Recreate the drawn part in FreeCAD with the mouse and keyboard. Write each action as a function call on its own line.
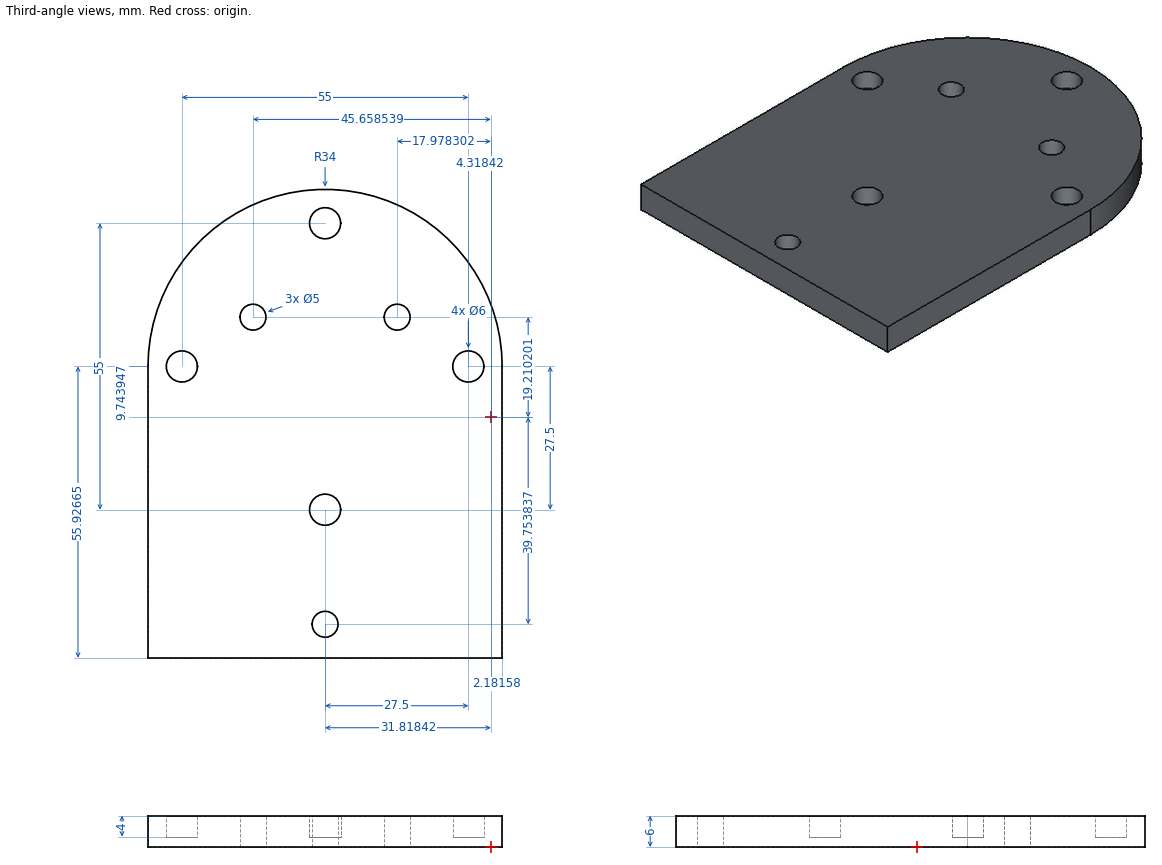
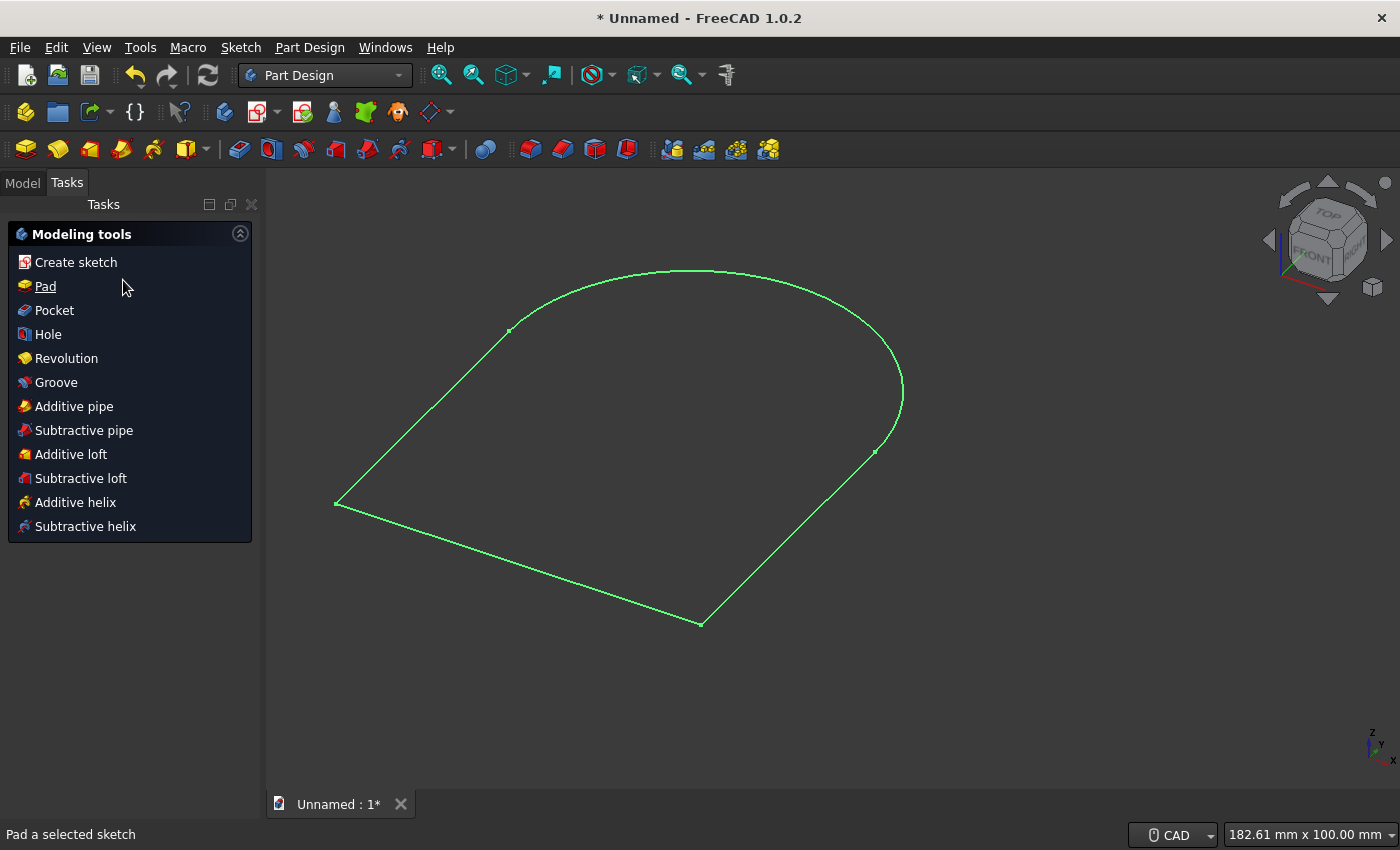
click(26, 150)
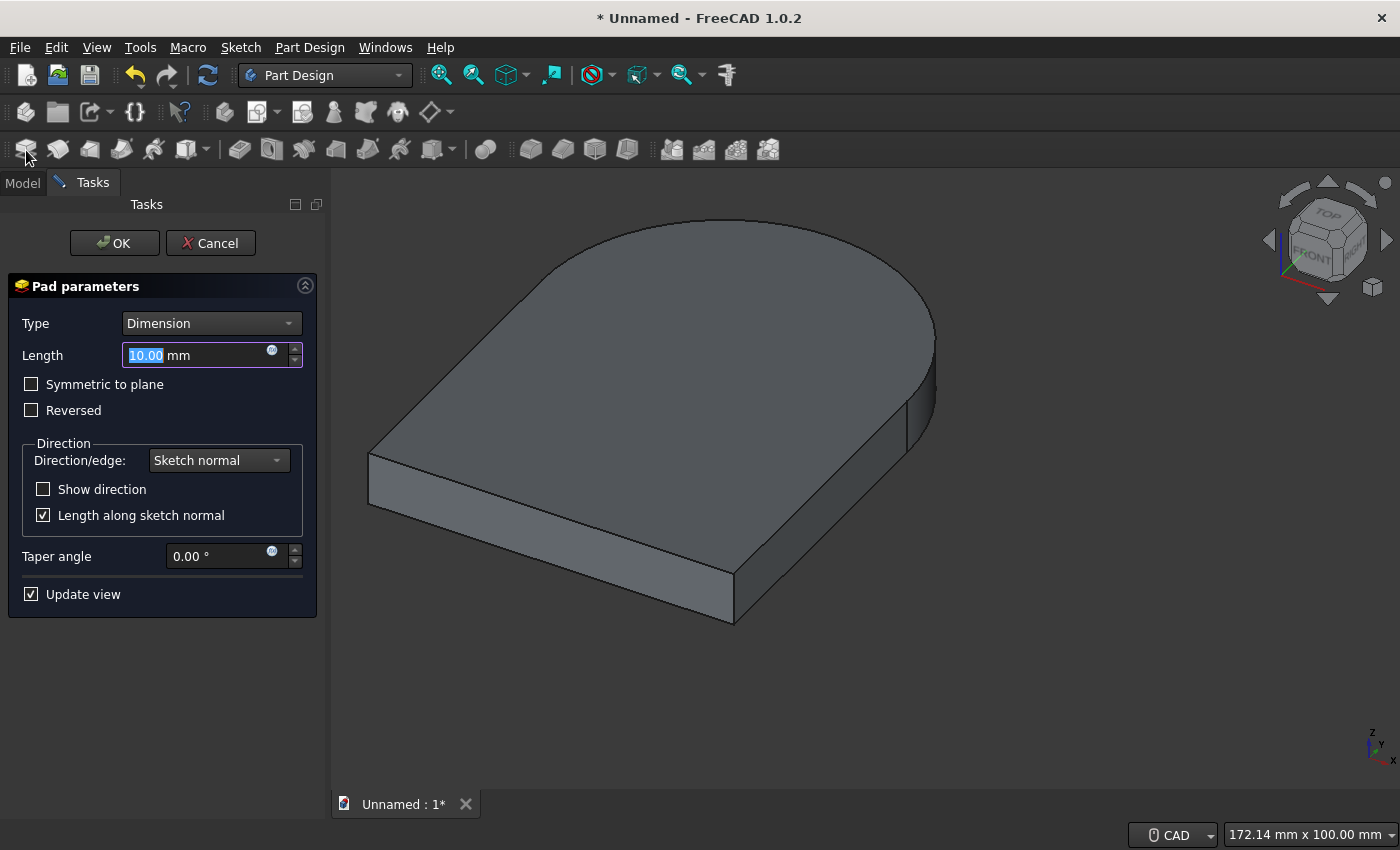
text(6)
key(Tab)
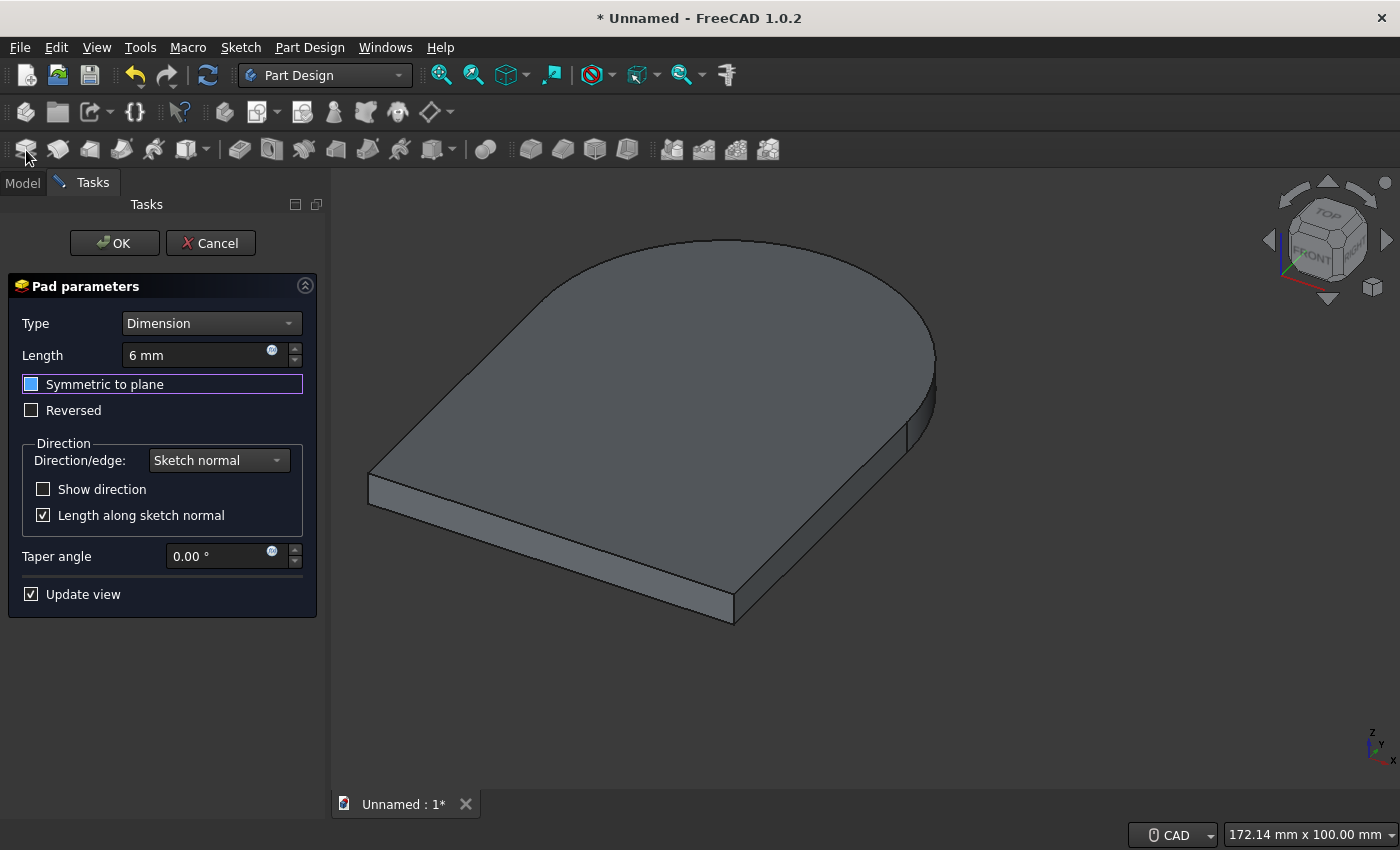
click(115, 243)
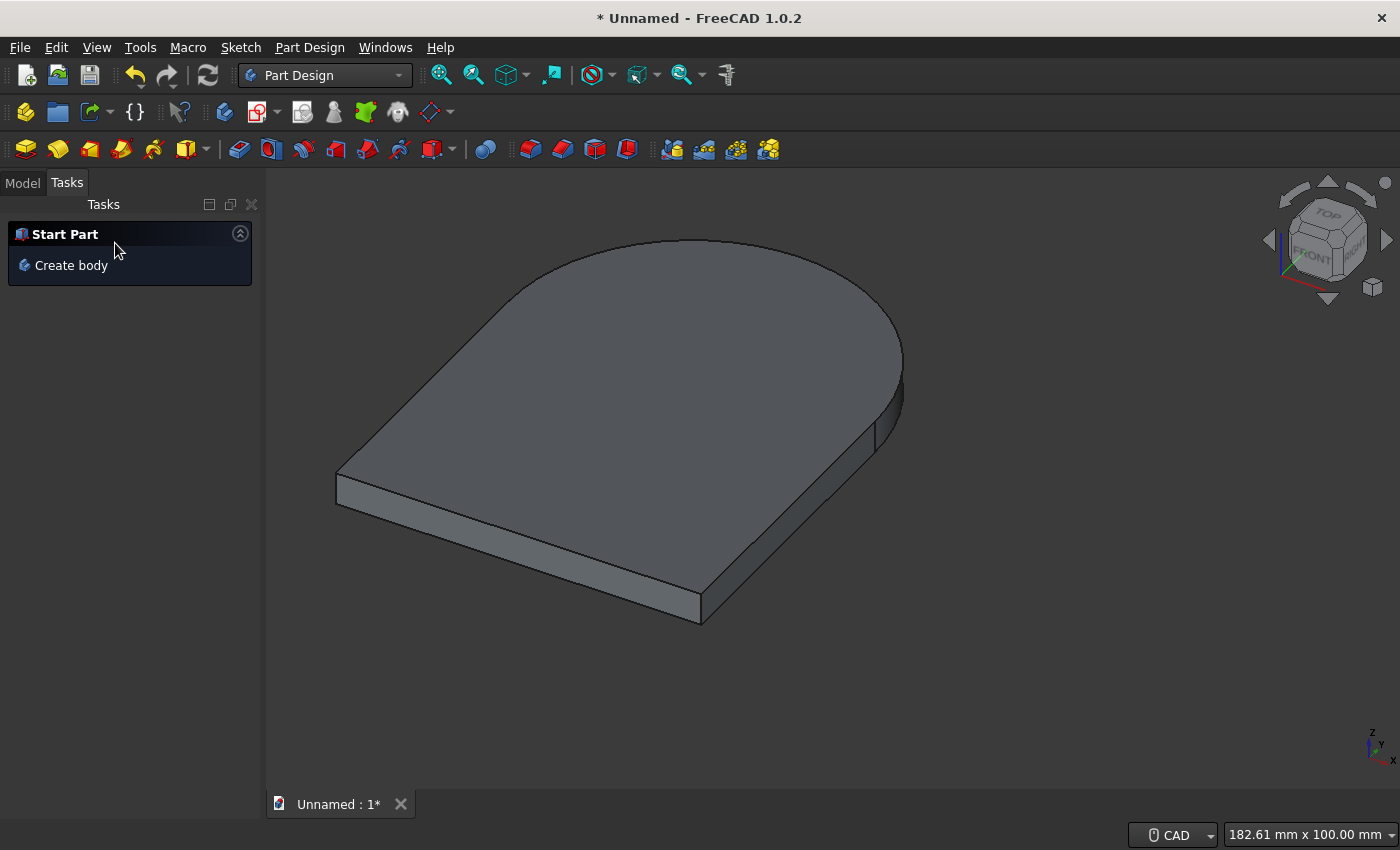
click(658, 394)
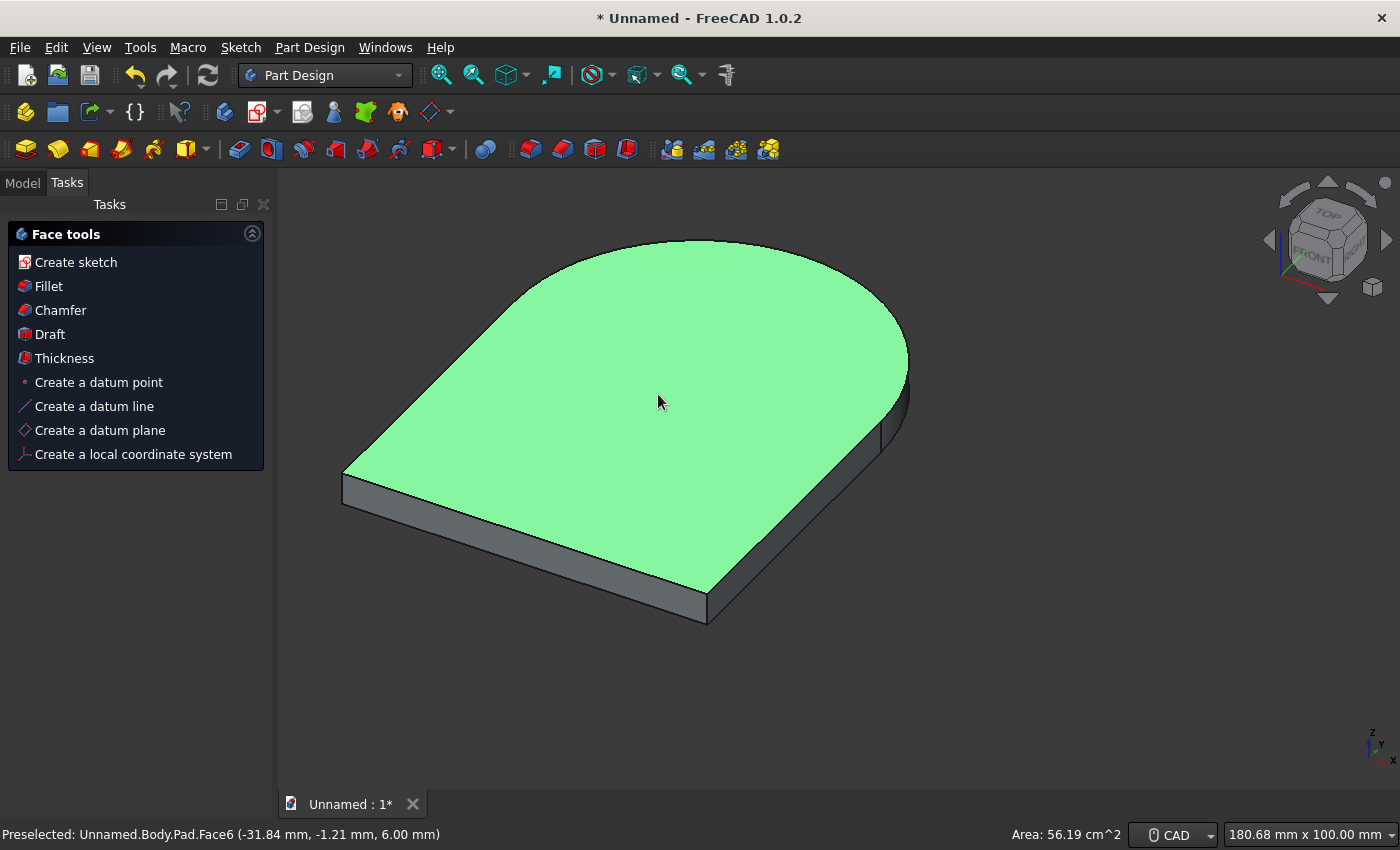
click(258, 112)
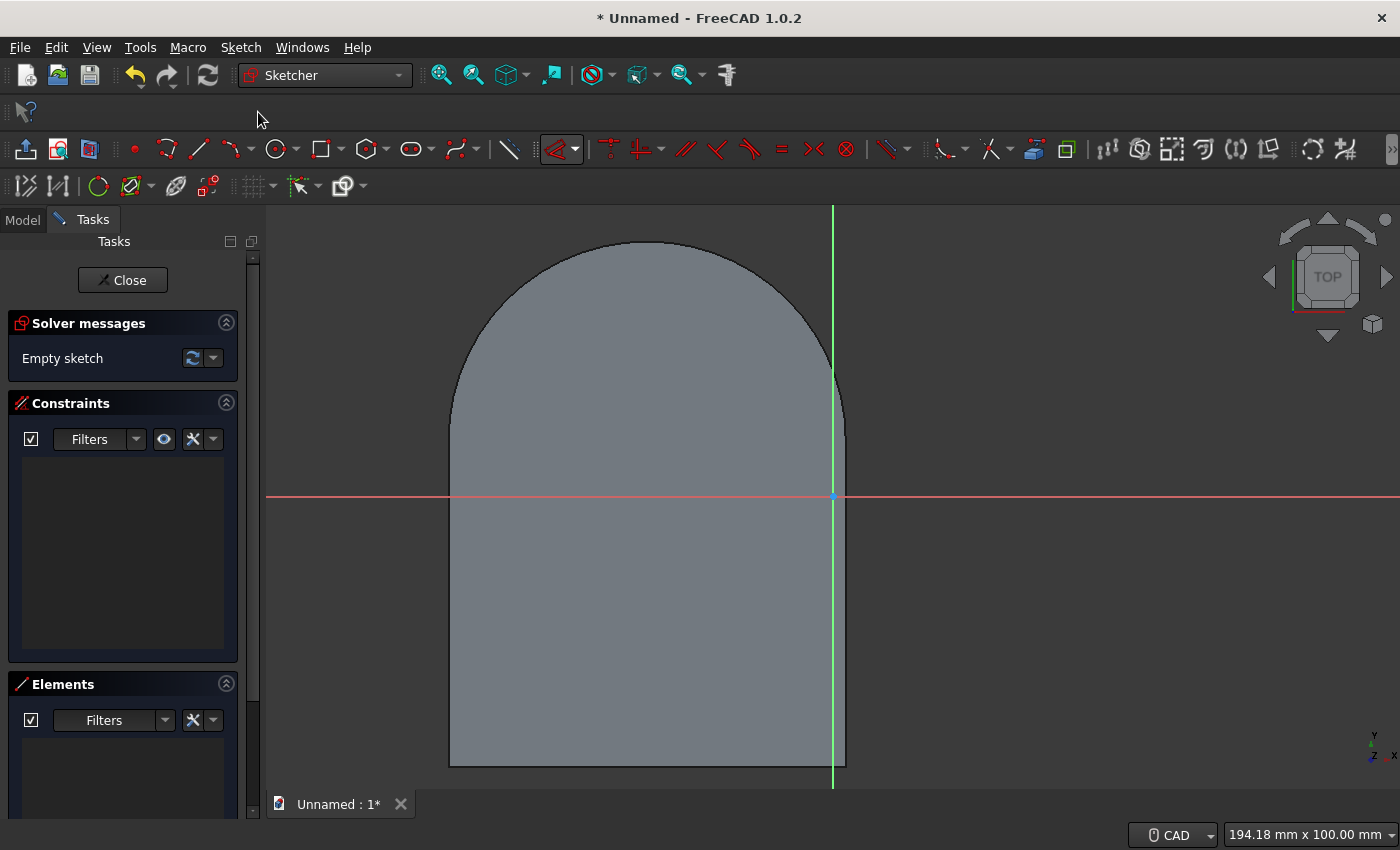
key(g)
key(c)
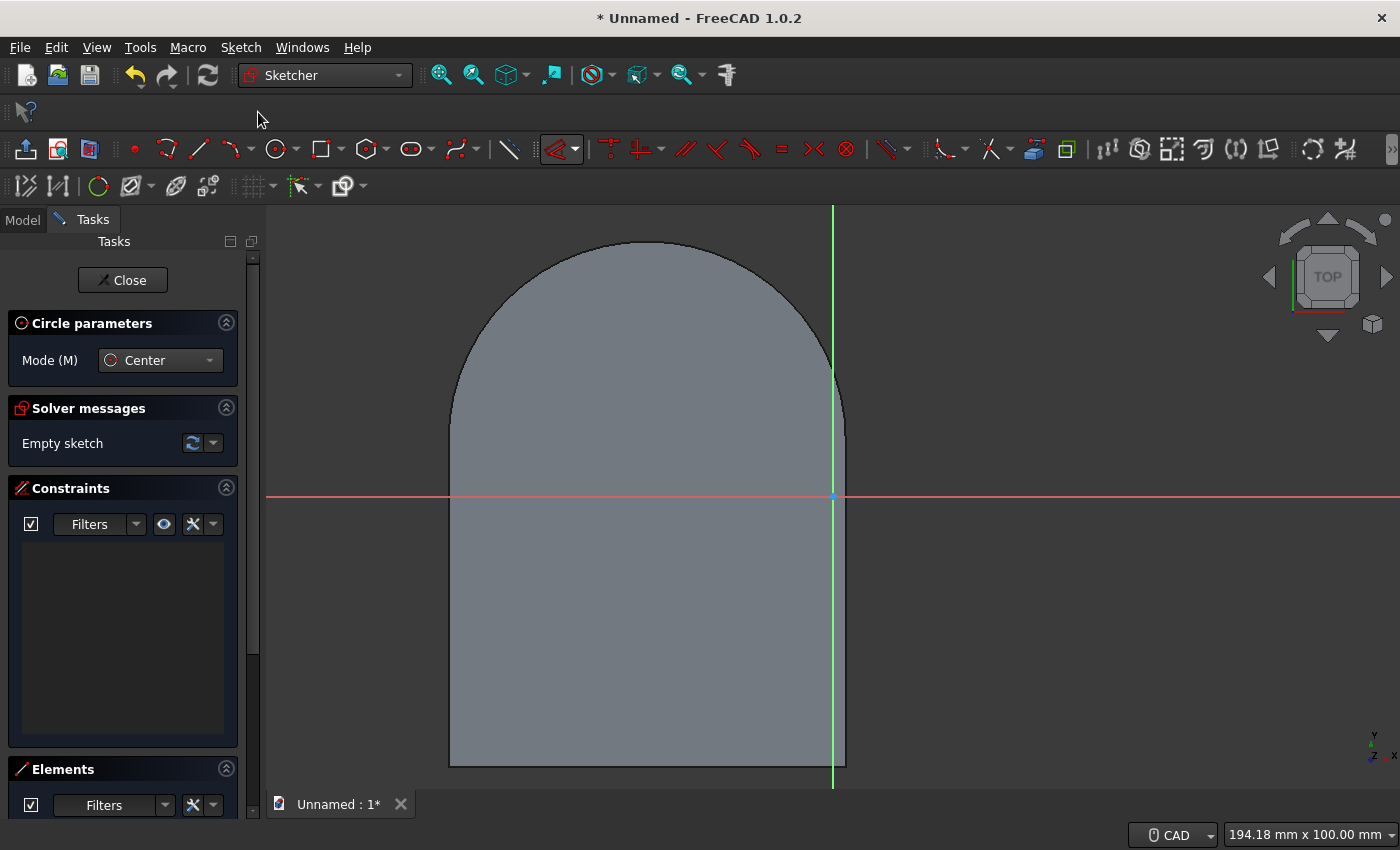
scroll(808, 440, up, 2)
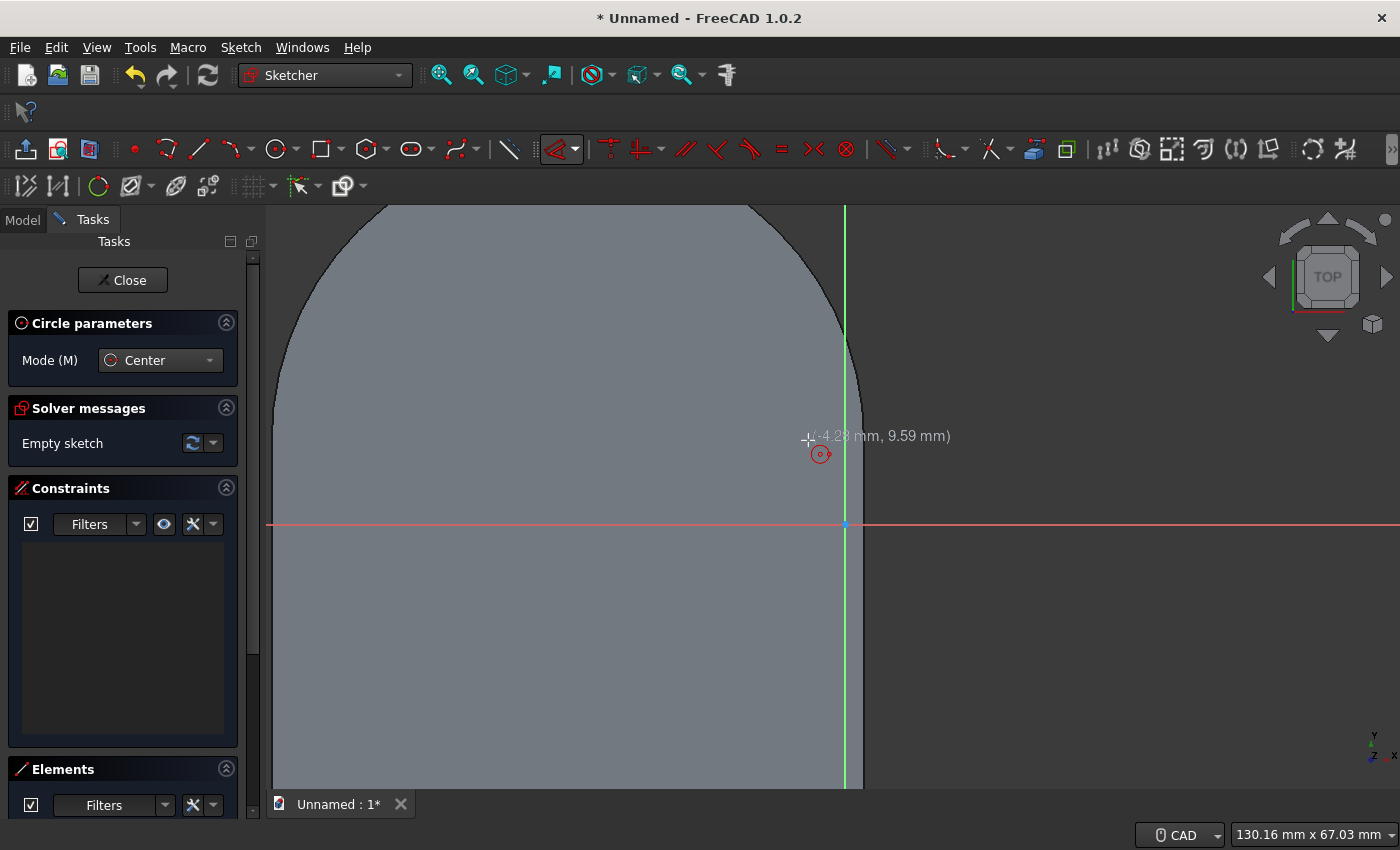
click(807, 440)
click(826, 421)